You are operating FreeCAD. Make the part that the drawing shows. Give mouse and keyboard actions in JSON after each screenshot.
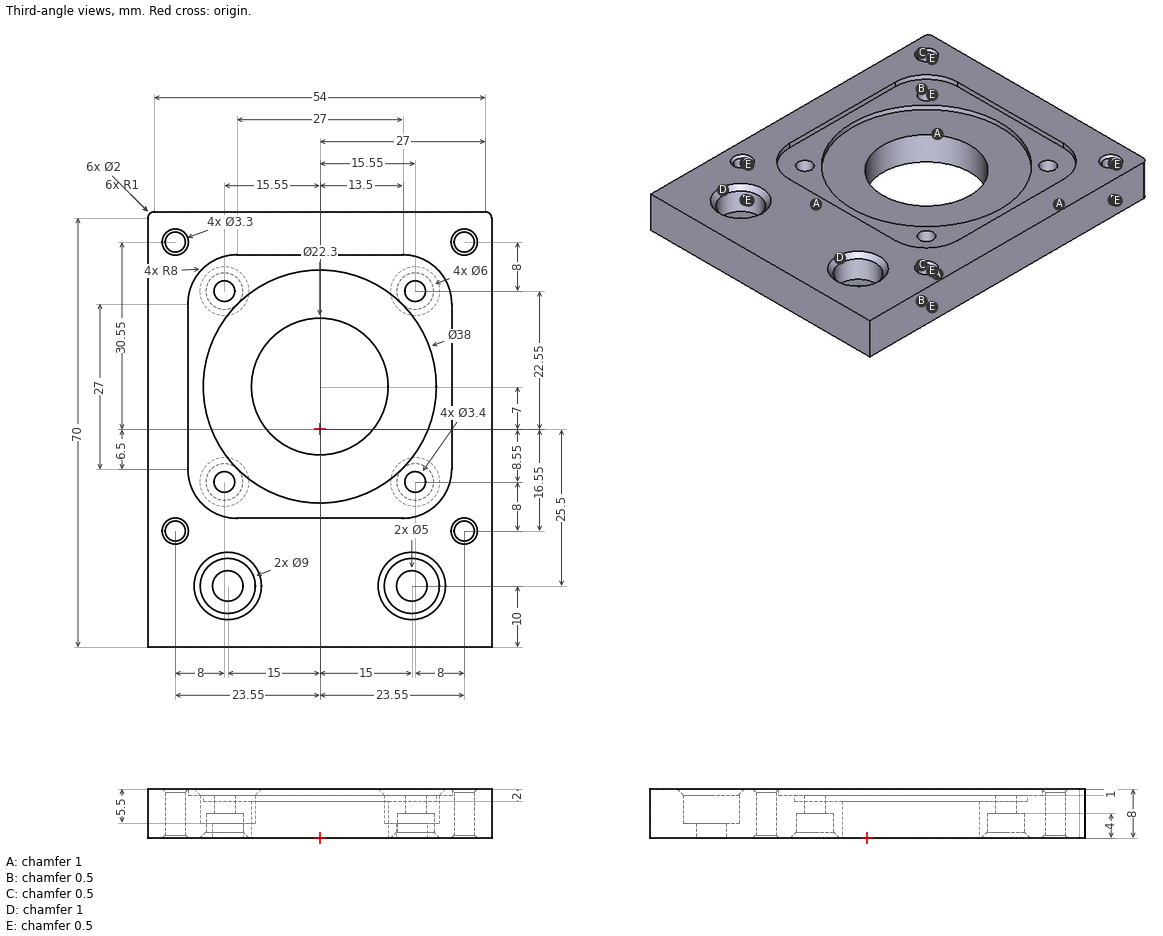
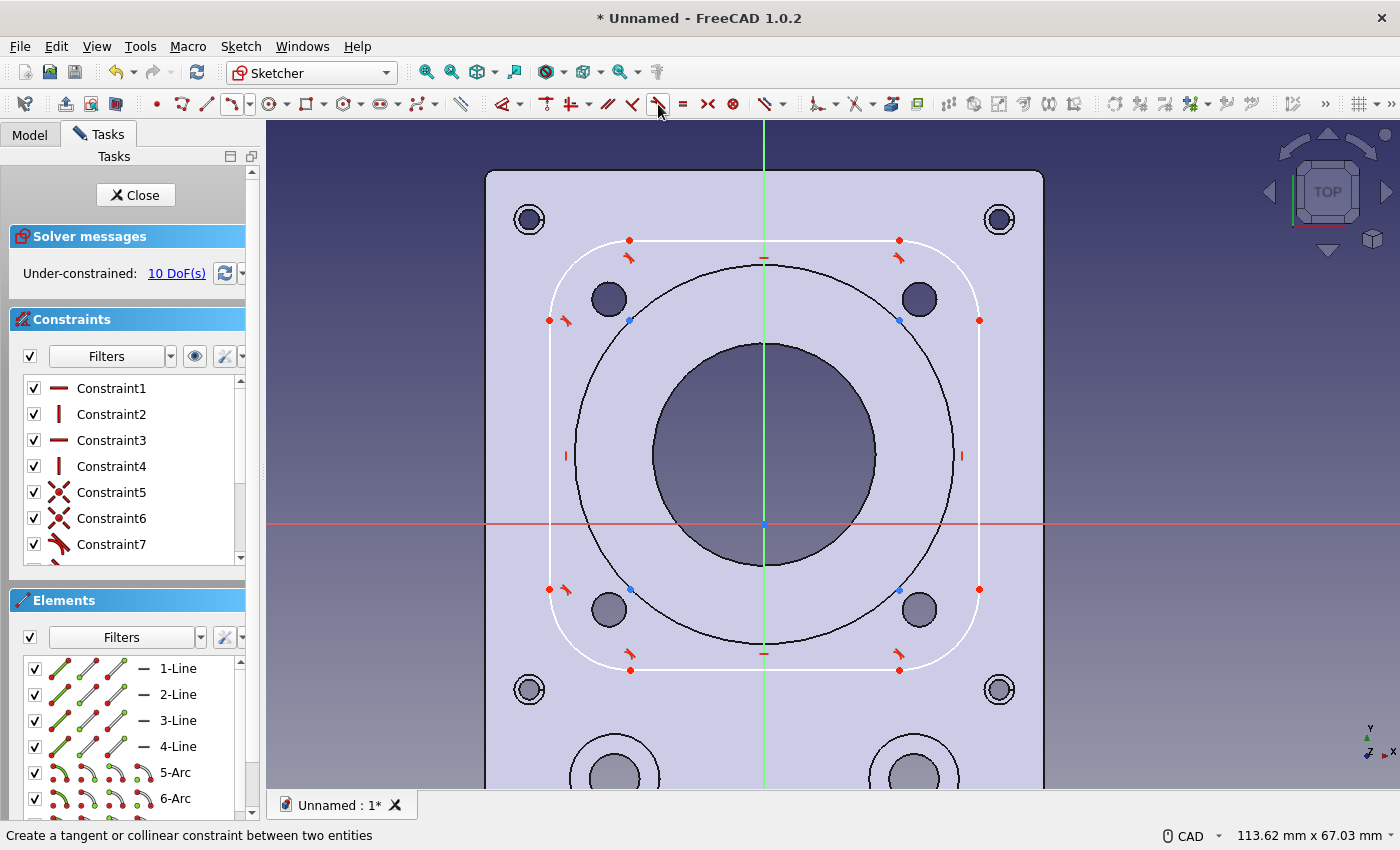
{"action": "left_click", "coordinate": [979, 509]}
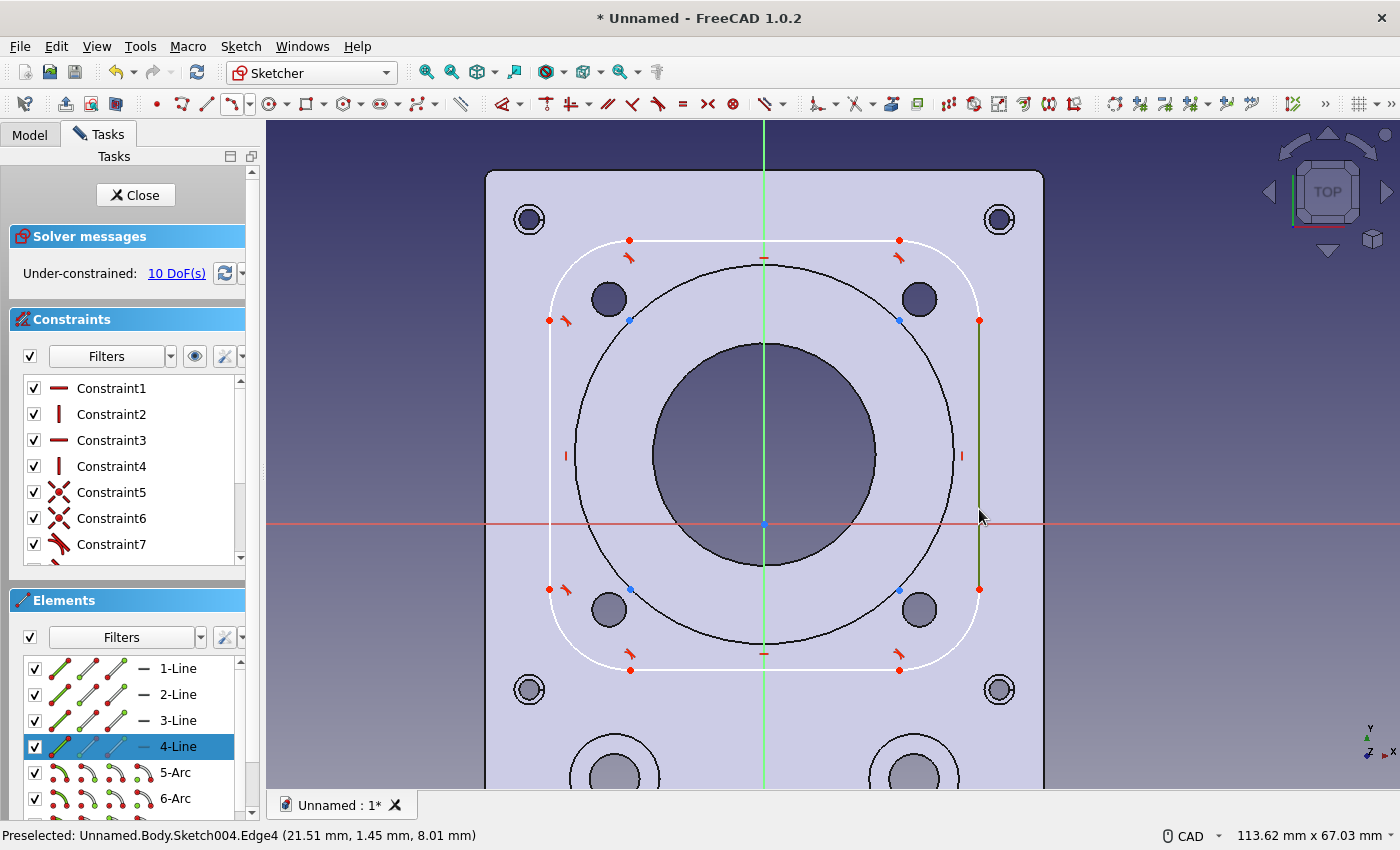
{"action": "left_click", "coordinate": [935, 661]}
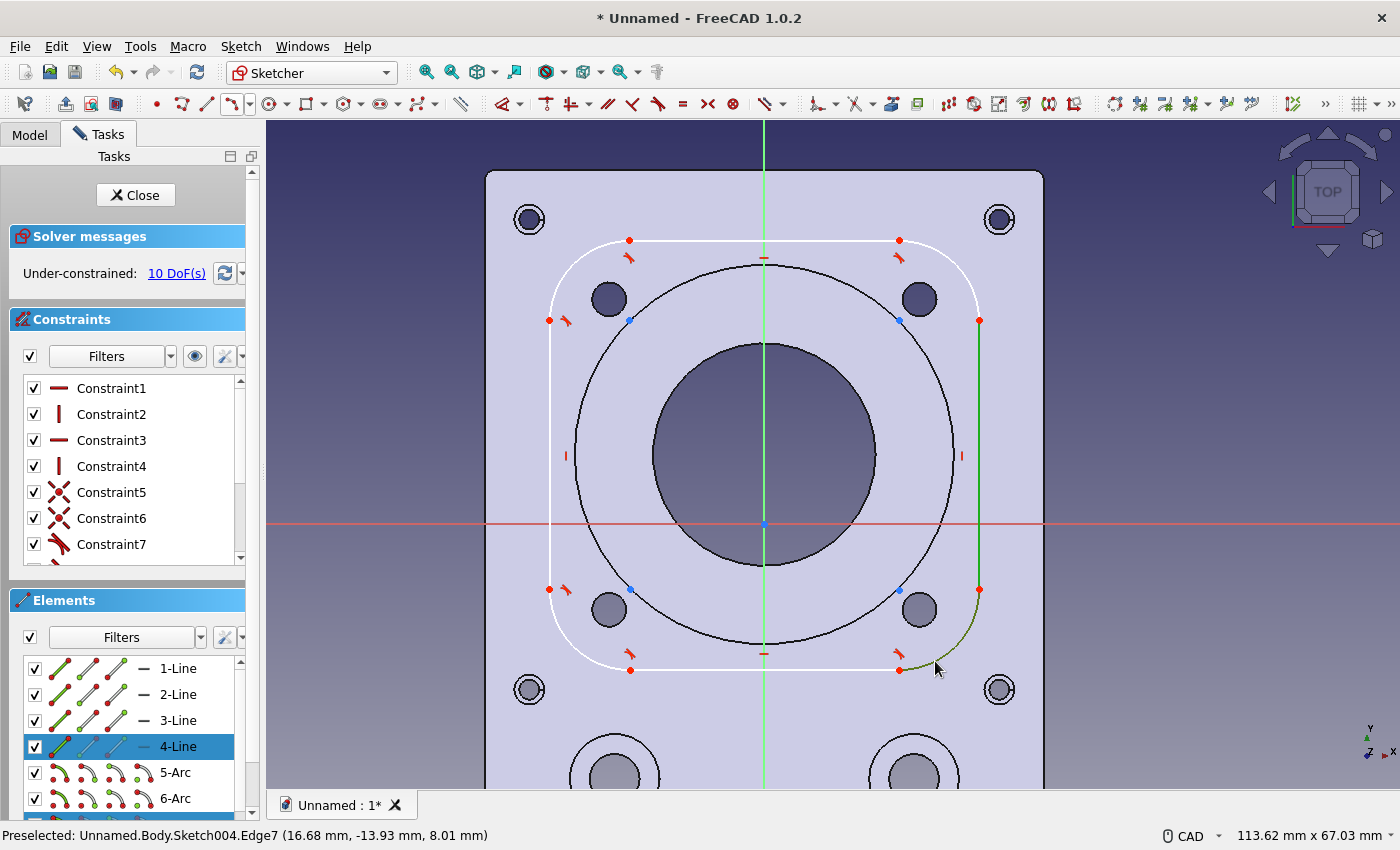
{"action": "key", "text": "t"}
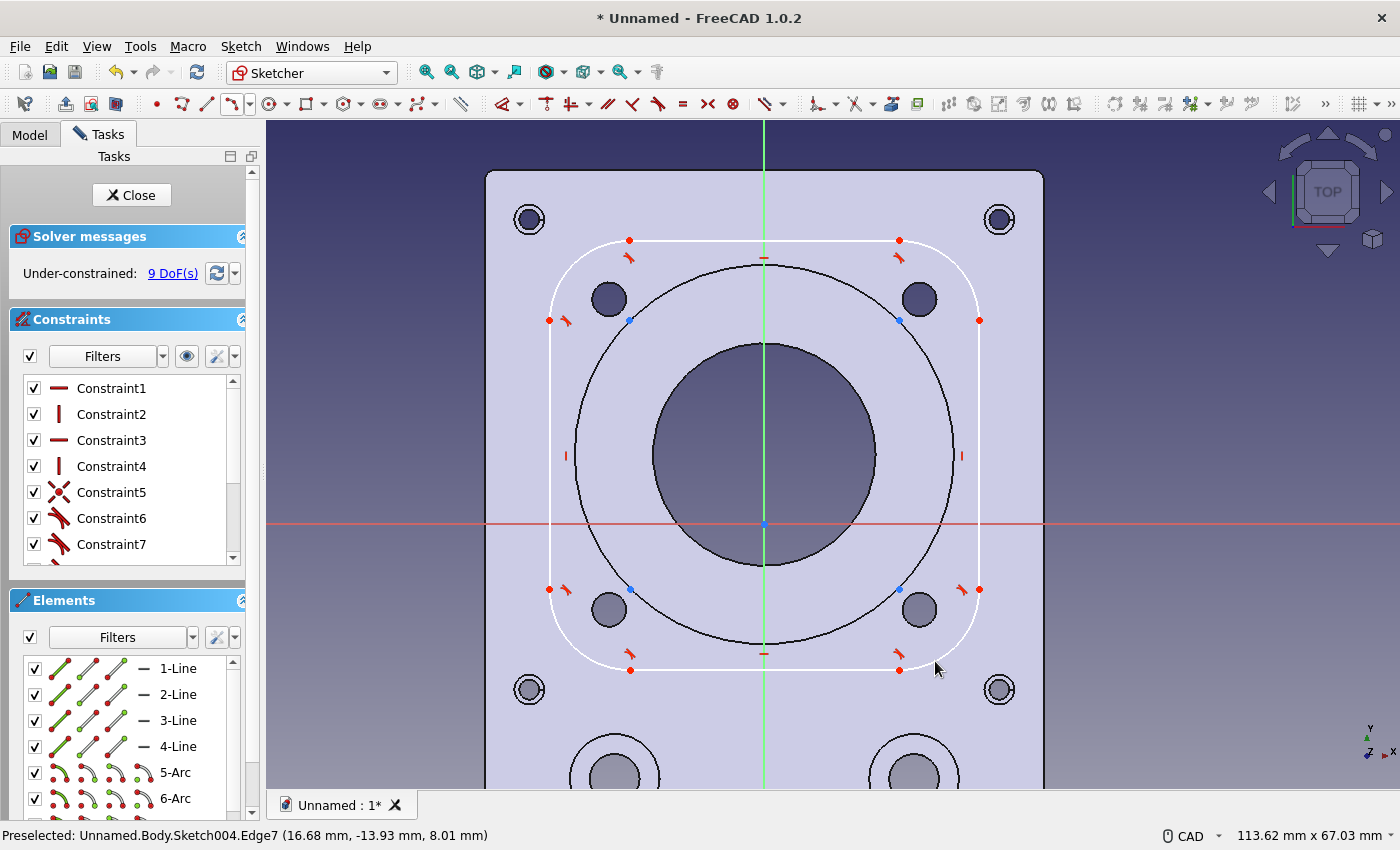
{"action": "left_click", "coordinate": [979, 509]}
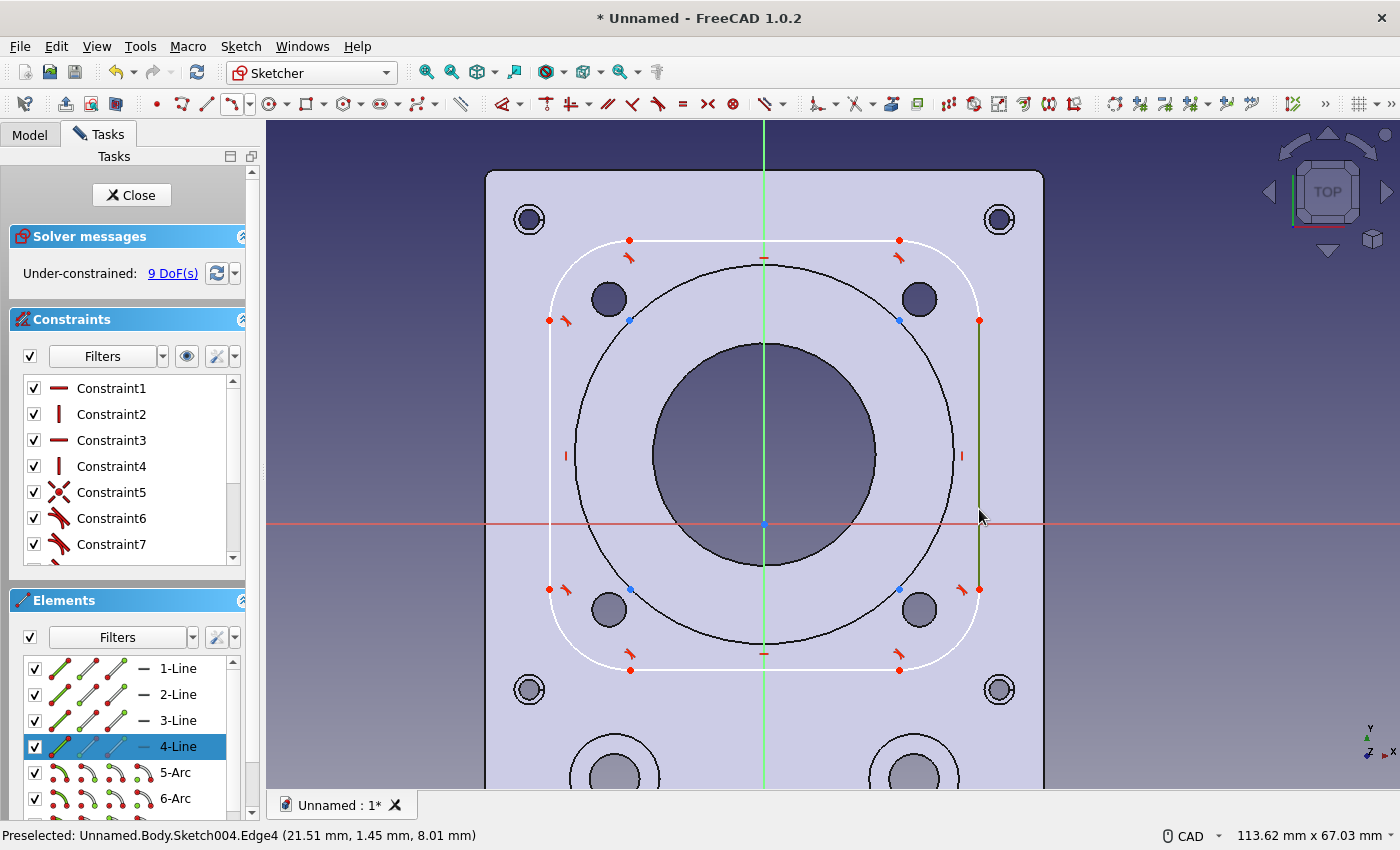
{"action": "left_click", "coordinate": [970, 285]}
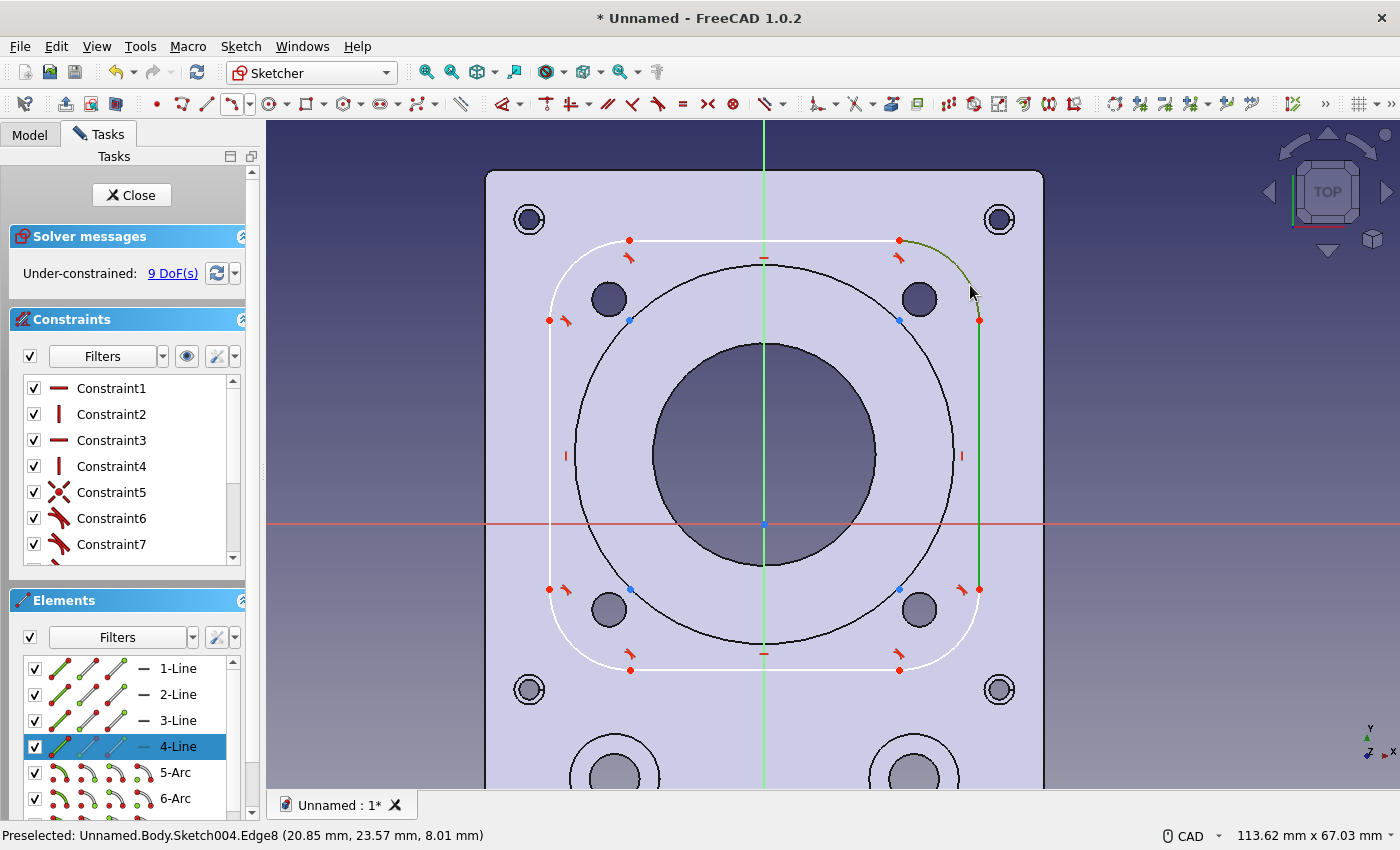
{"action": "key", "text": "t"}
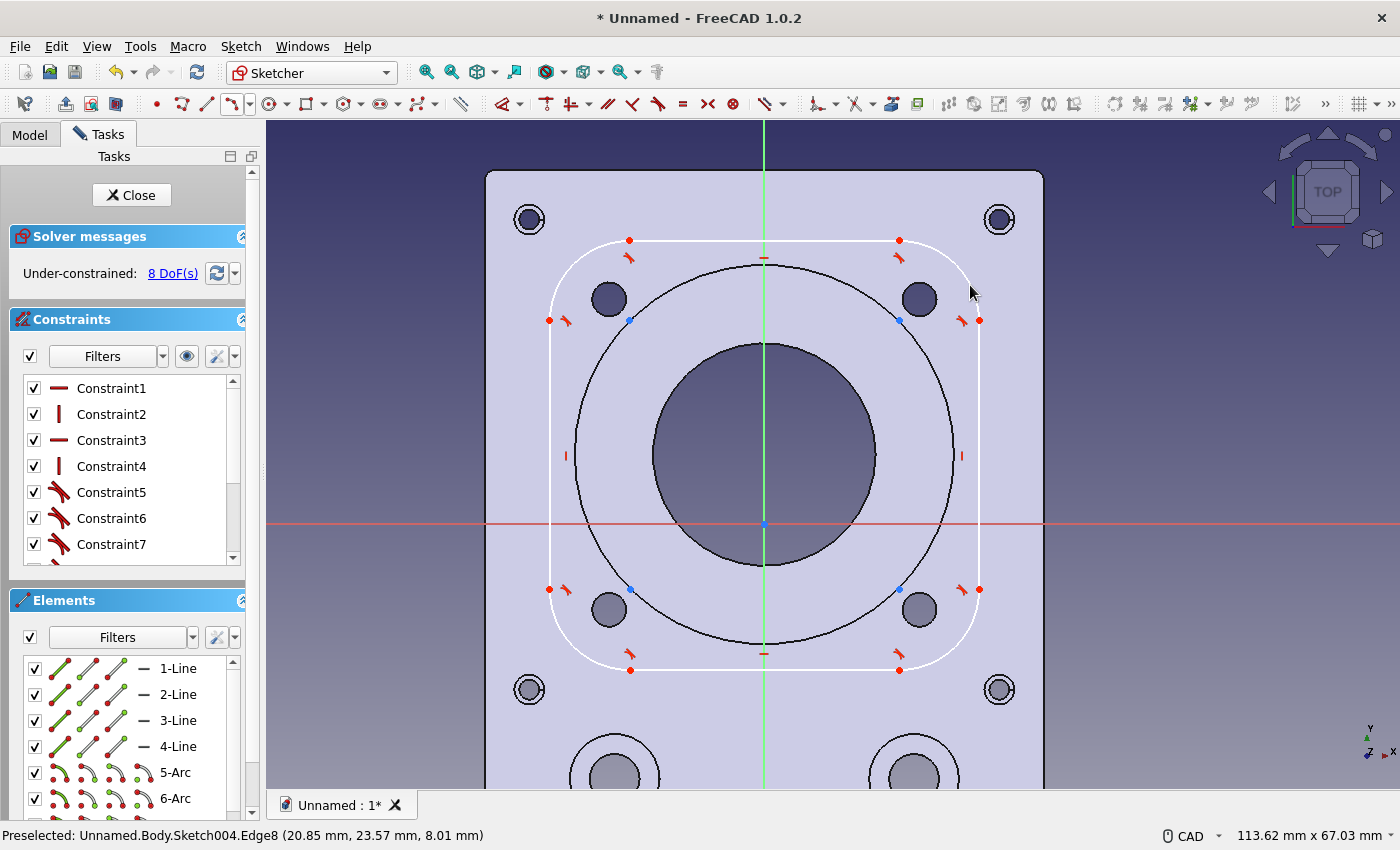
{"action": "left_click", "coordinate": [594, 250]}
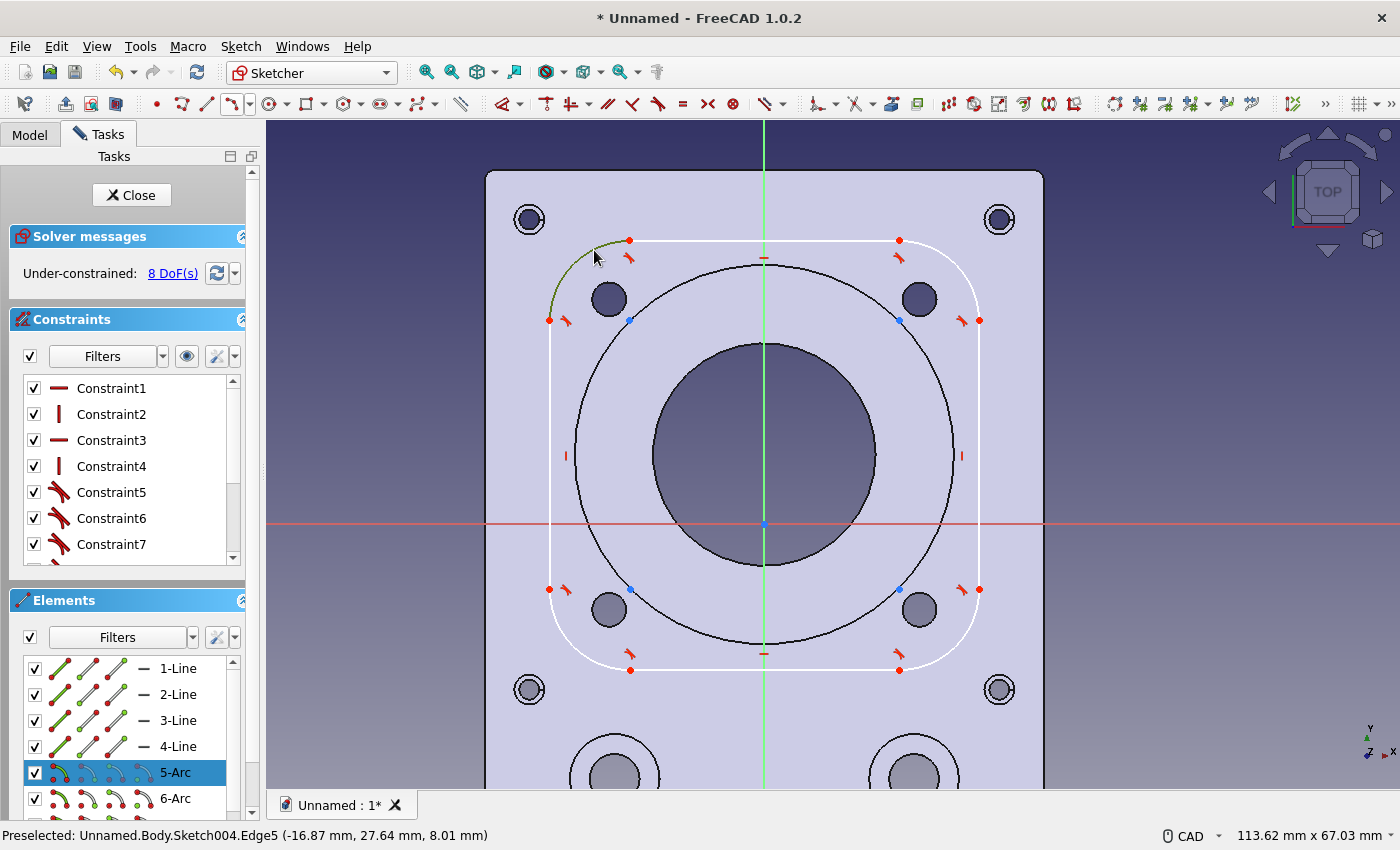
{"action": "left_click", "coordinate": [559, 626]}